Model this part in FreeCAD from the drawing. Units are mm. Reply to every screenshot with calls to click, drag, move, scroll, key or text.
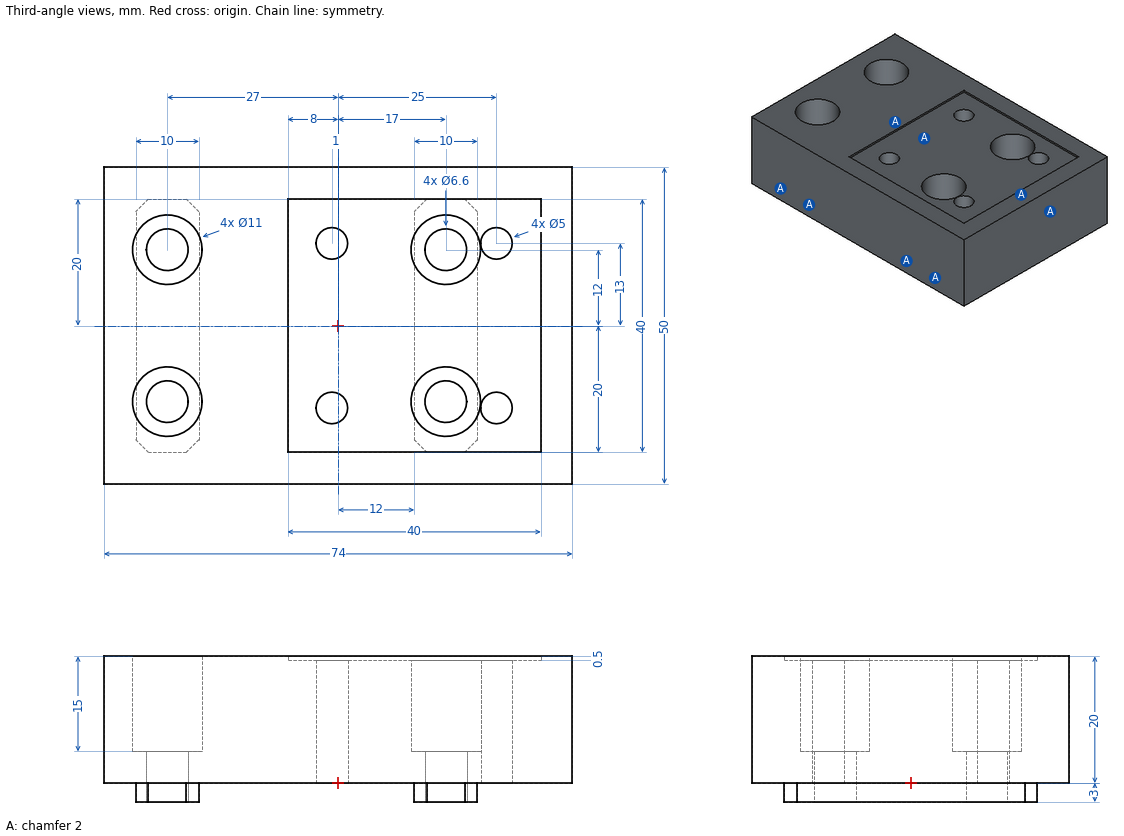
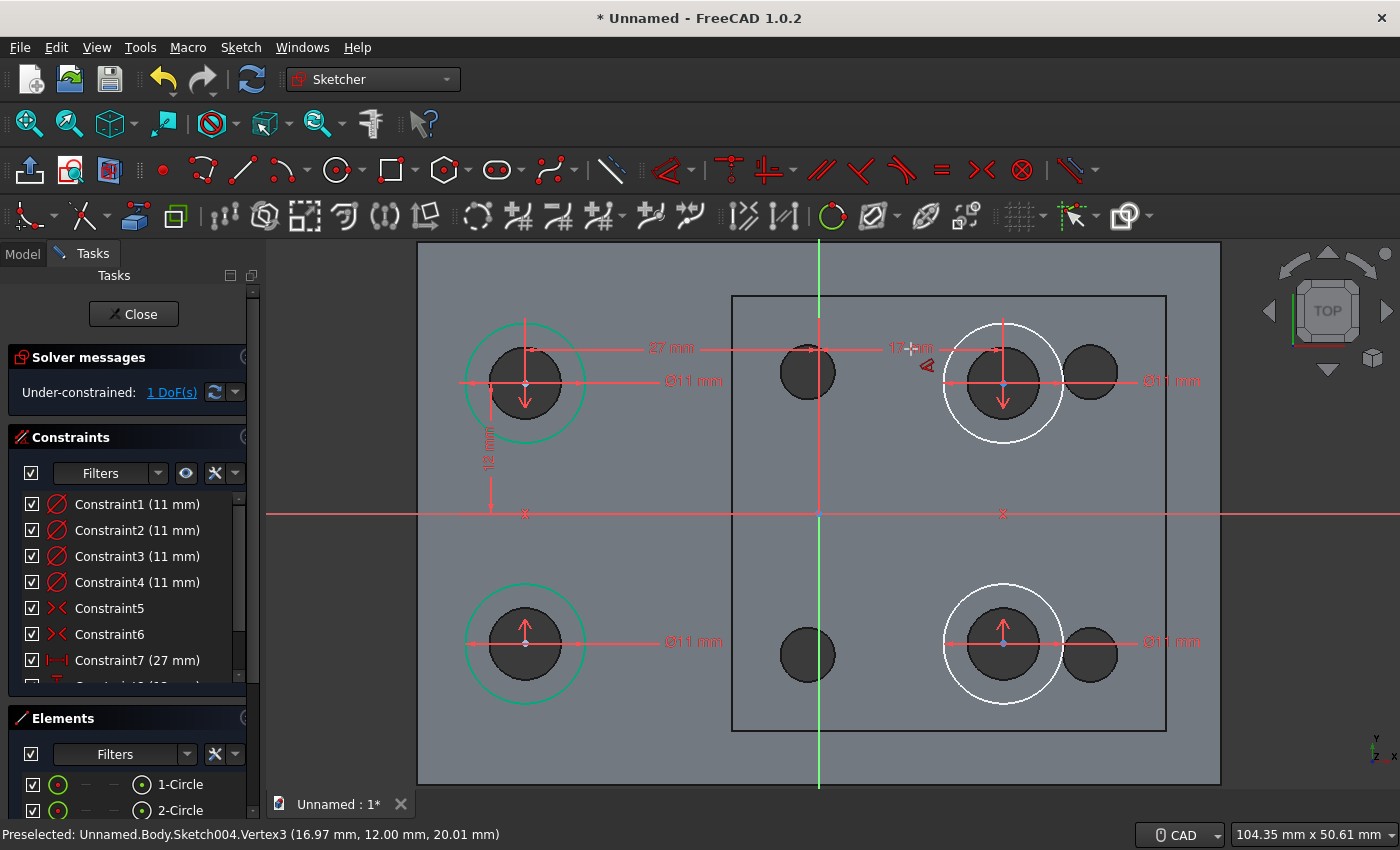
click(1003, 383)
click(1037, 448)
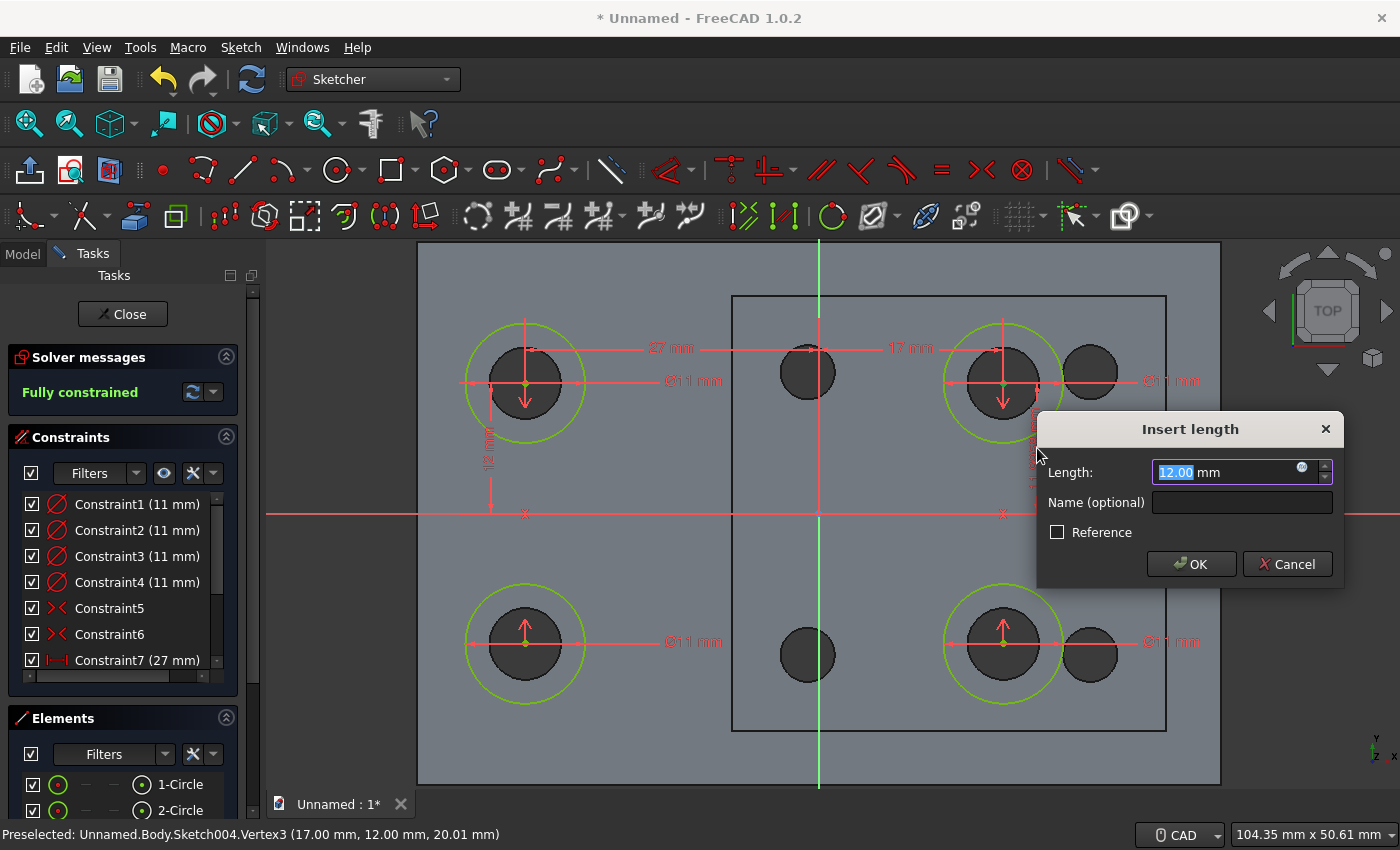
text(12)
key(Return)
key(Escape)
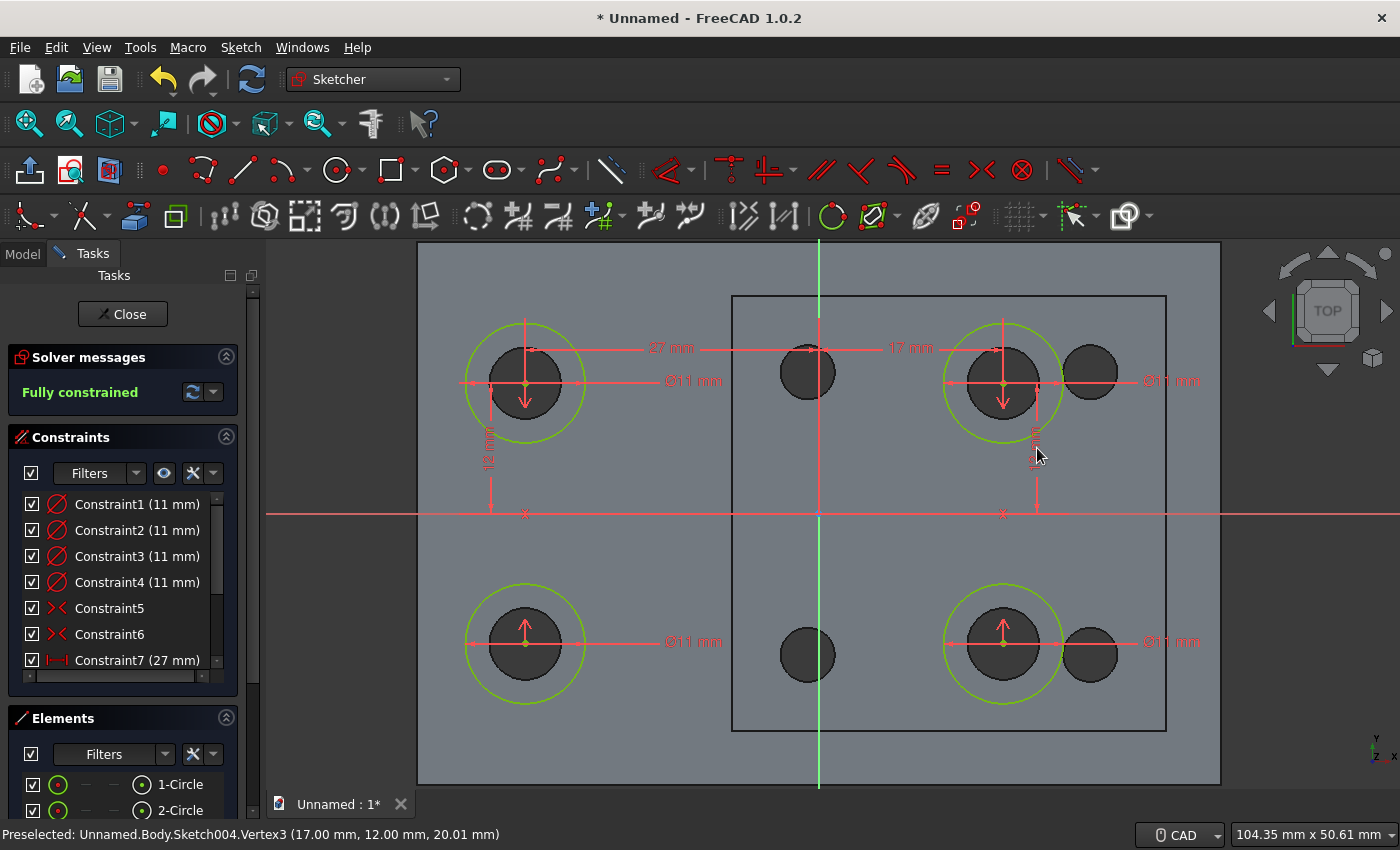
click(123, 314)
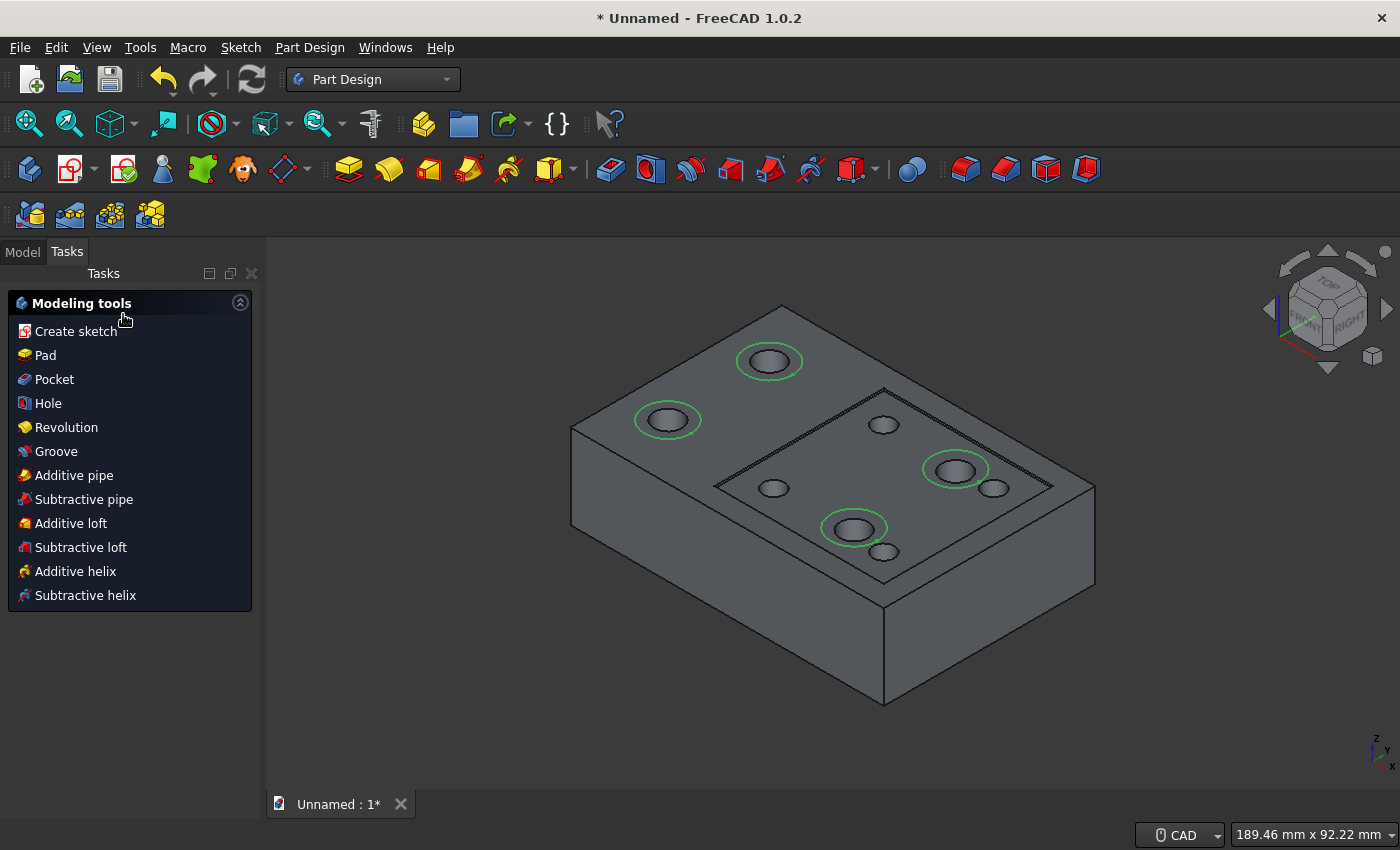
click(612, 170)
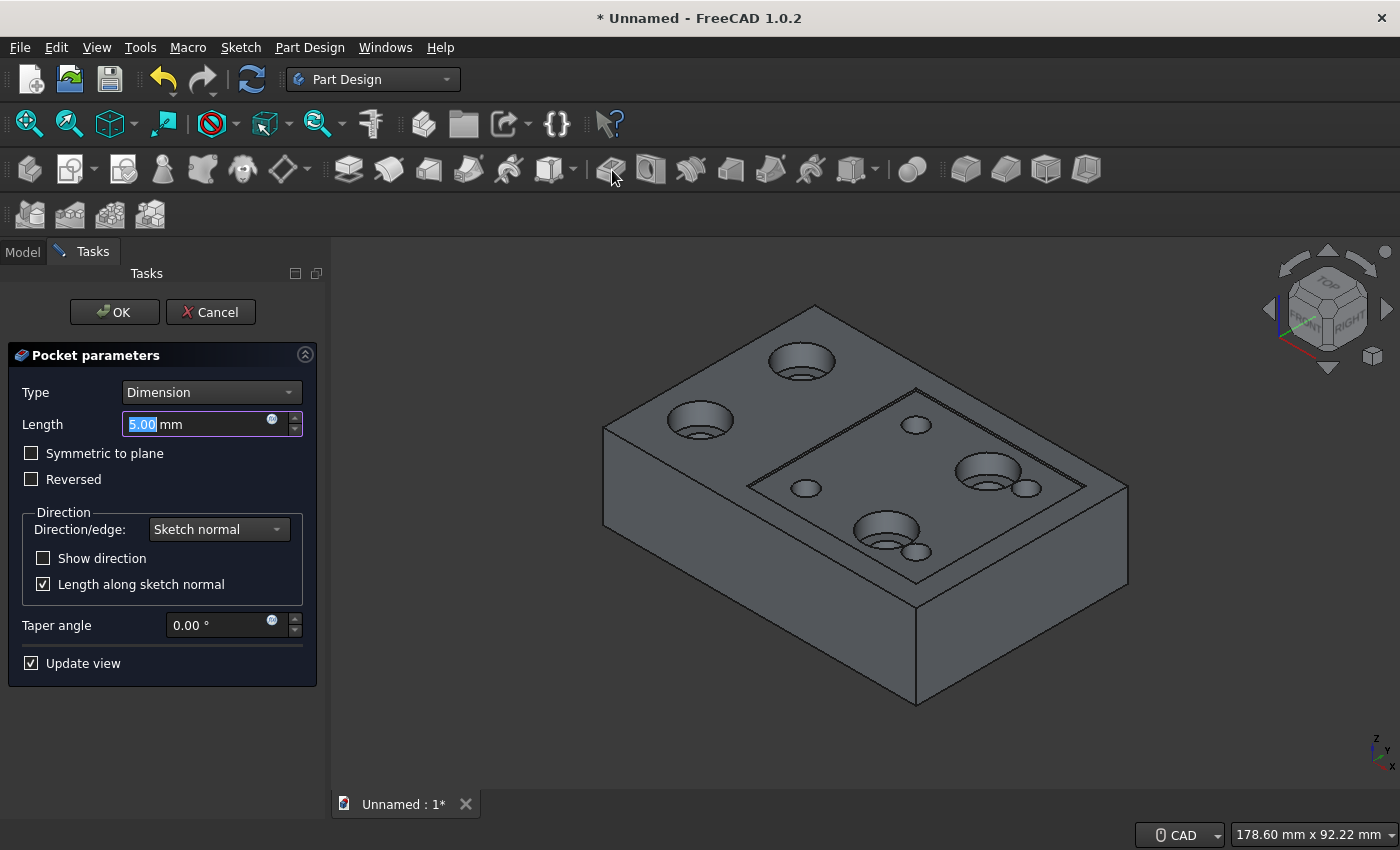
text(15)
key(Tab)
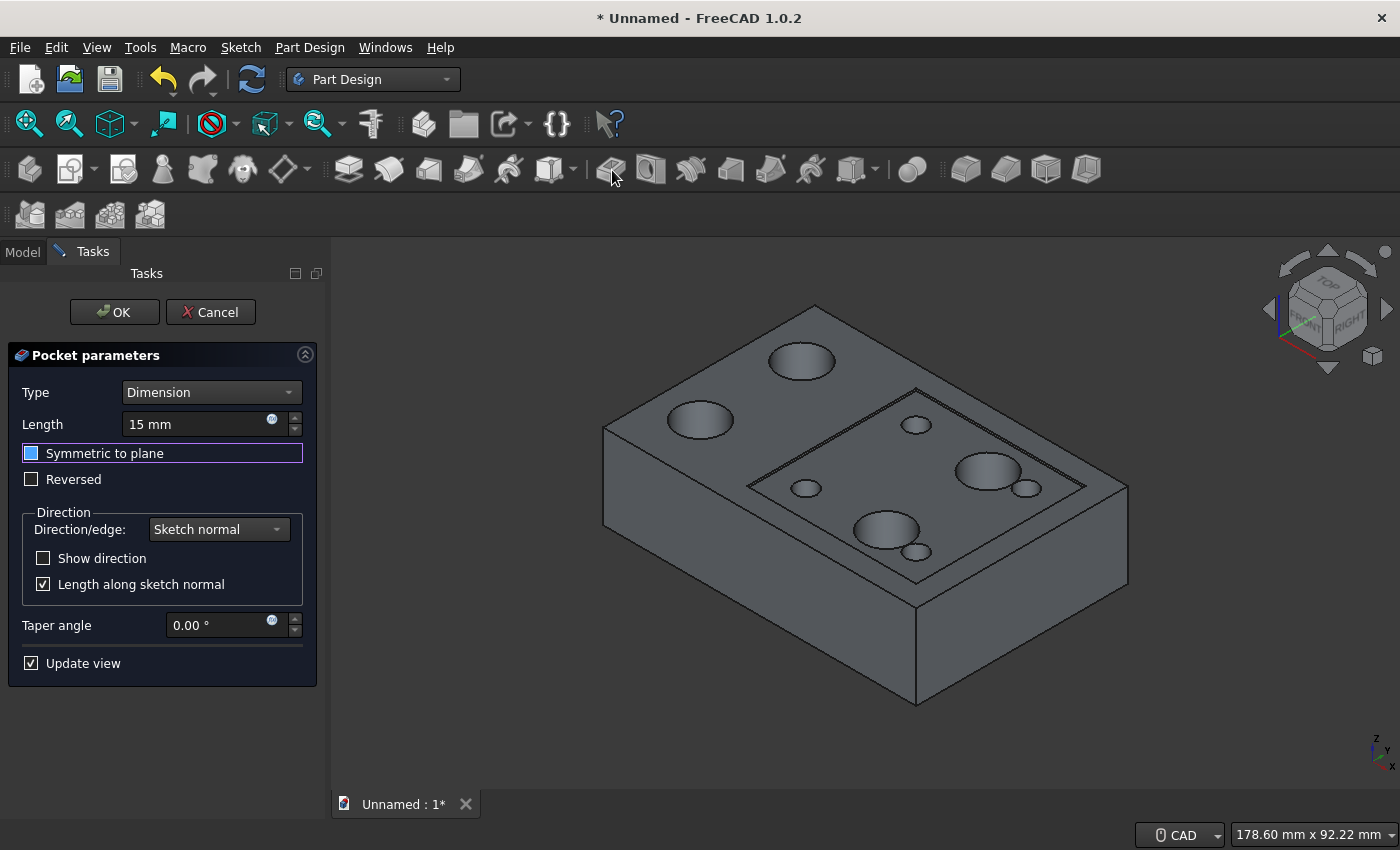
click(115, 312)